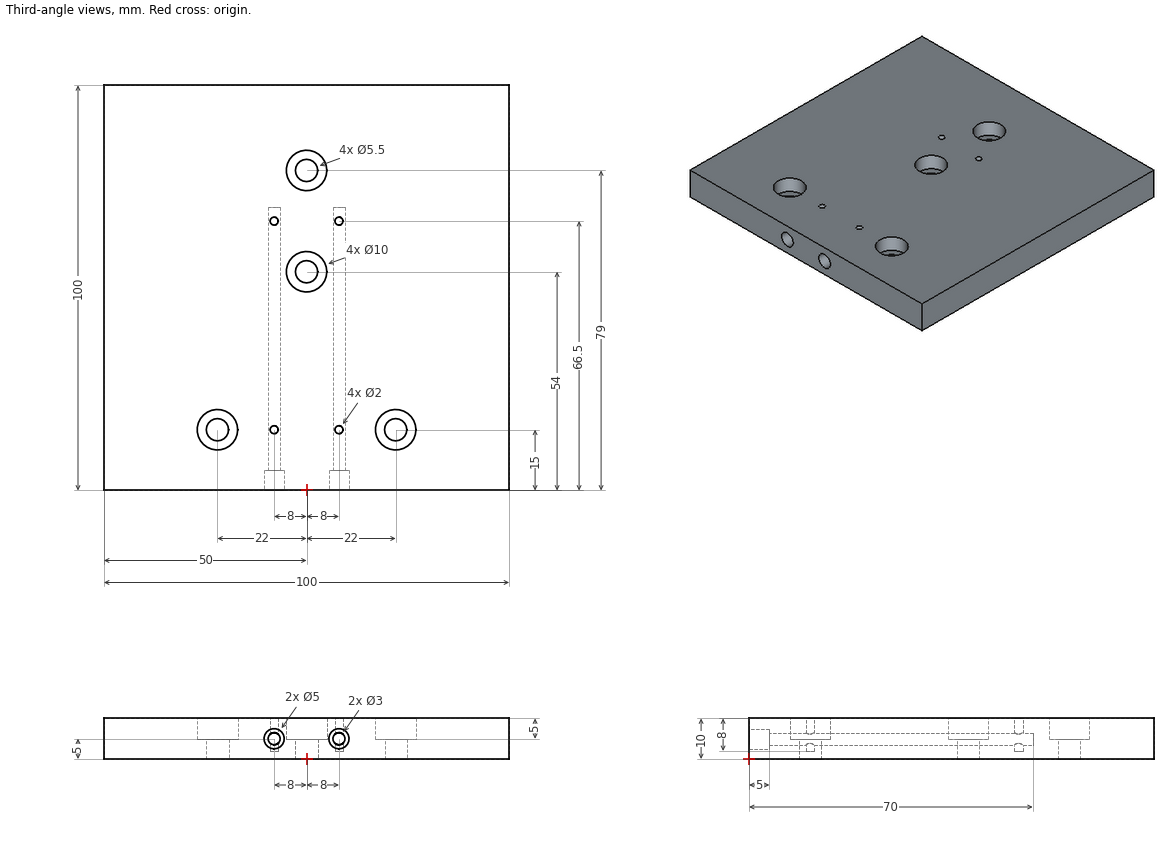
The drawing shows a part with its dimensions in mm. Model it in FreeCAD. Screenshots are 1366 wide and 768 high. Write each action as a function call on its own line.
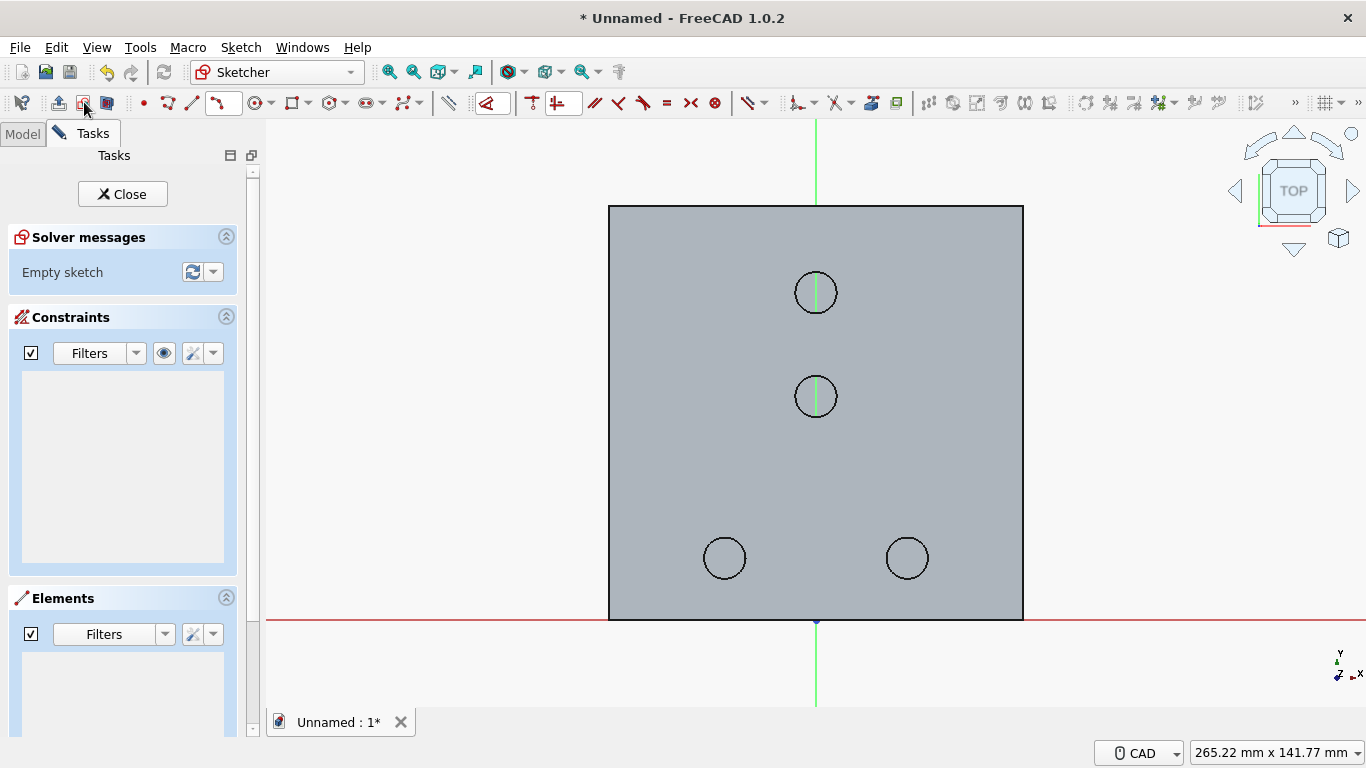
click(108, 104)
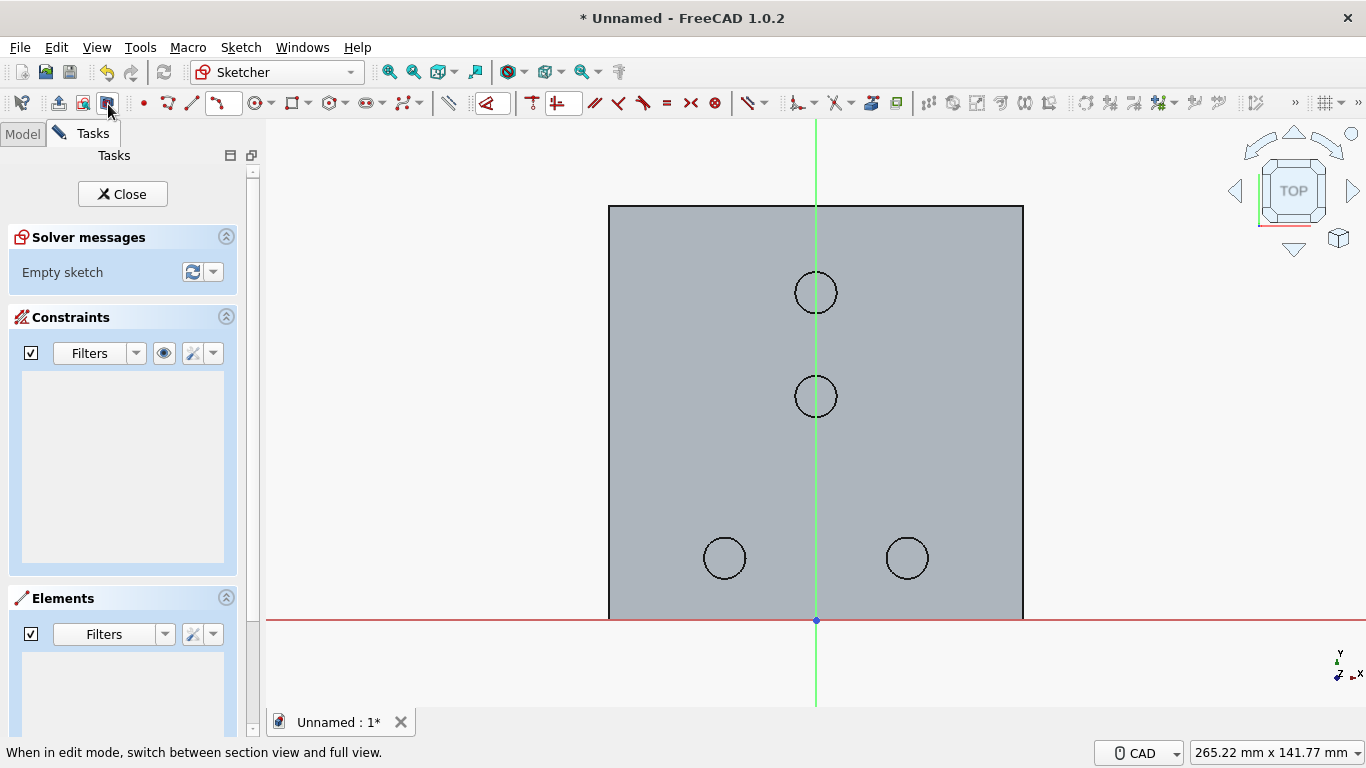
click(256, 104)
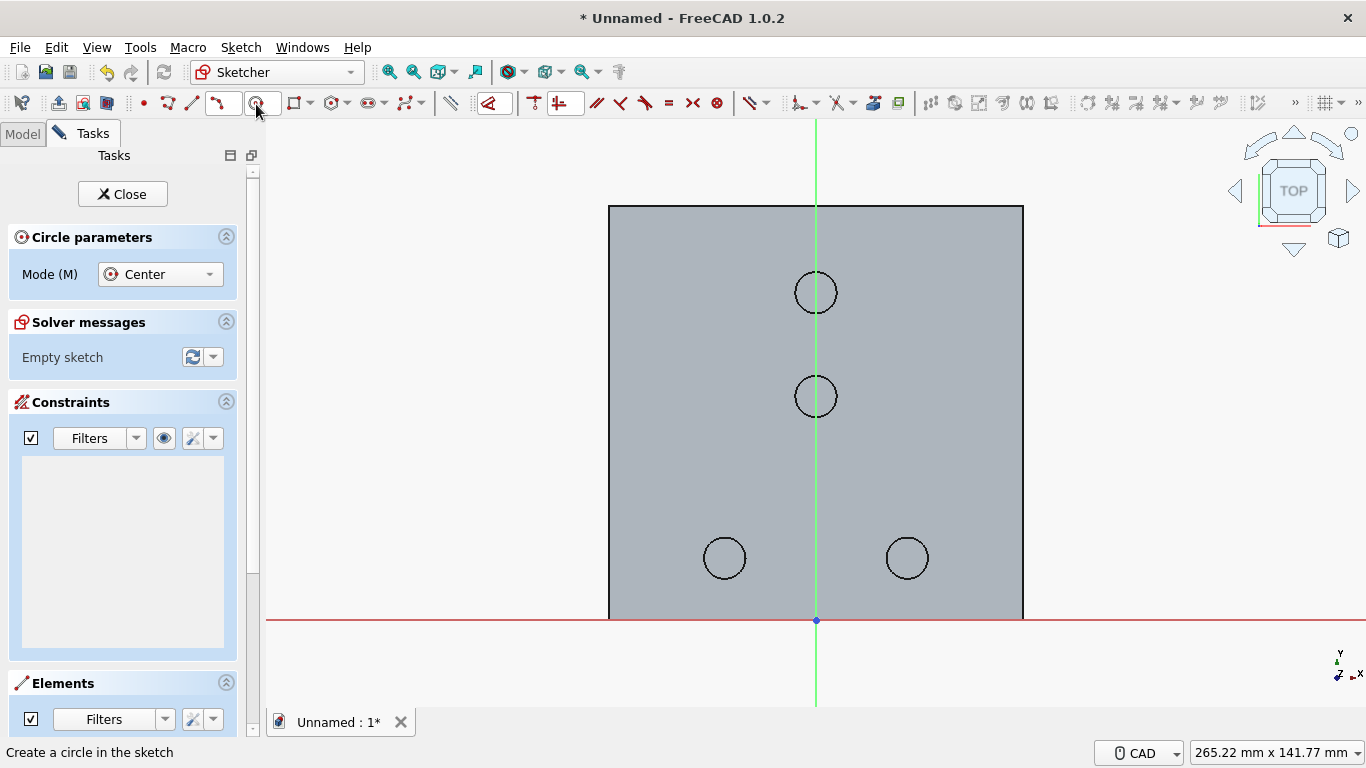
scroll(816, 293, up, 4)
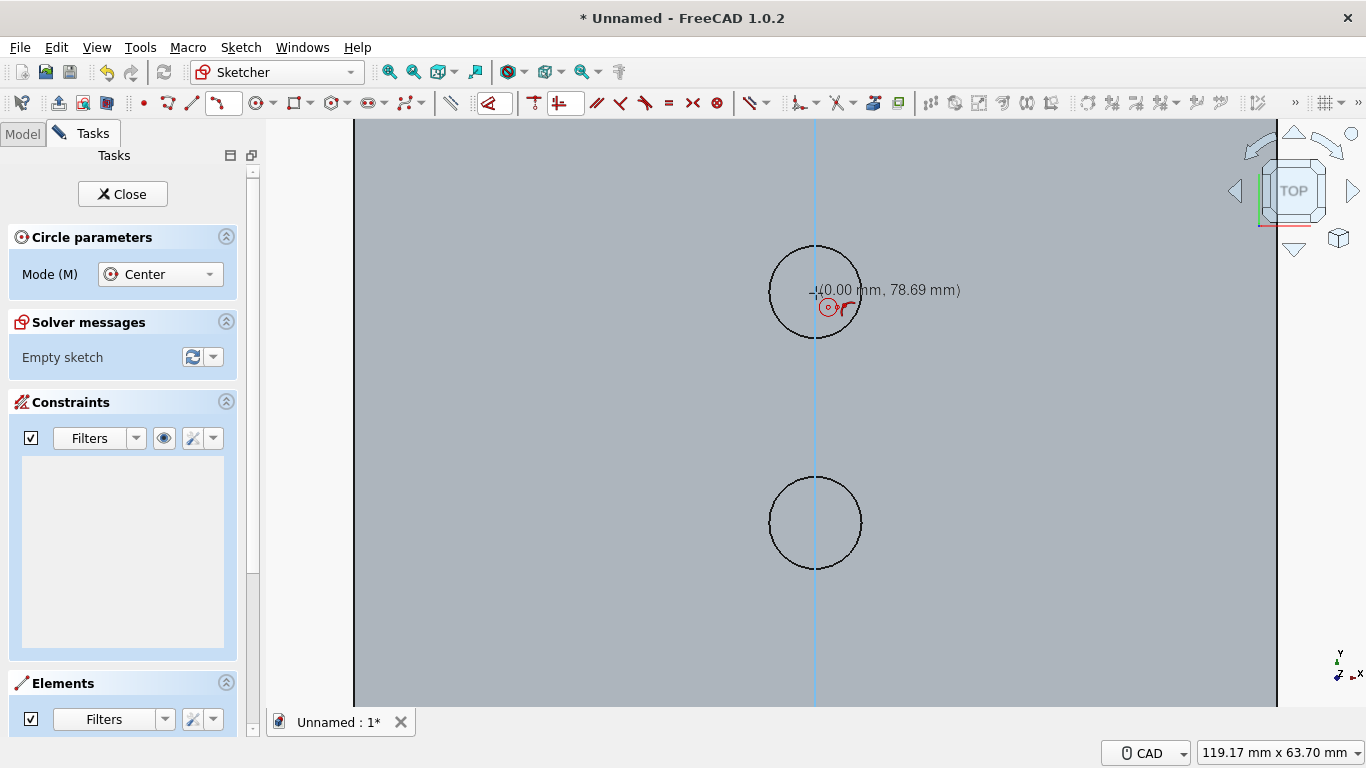
click(815, 292)
click(833, 274)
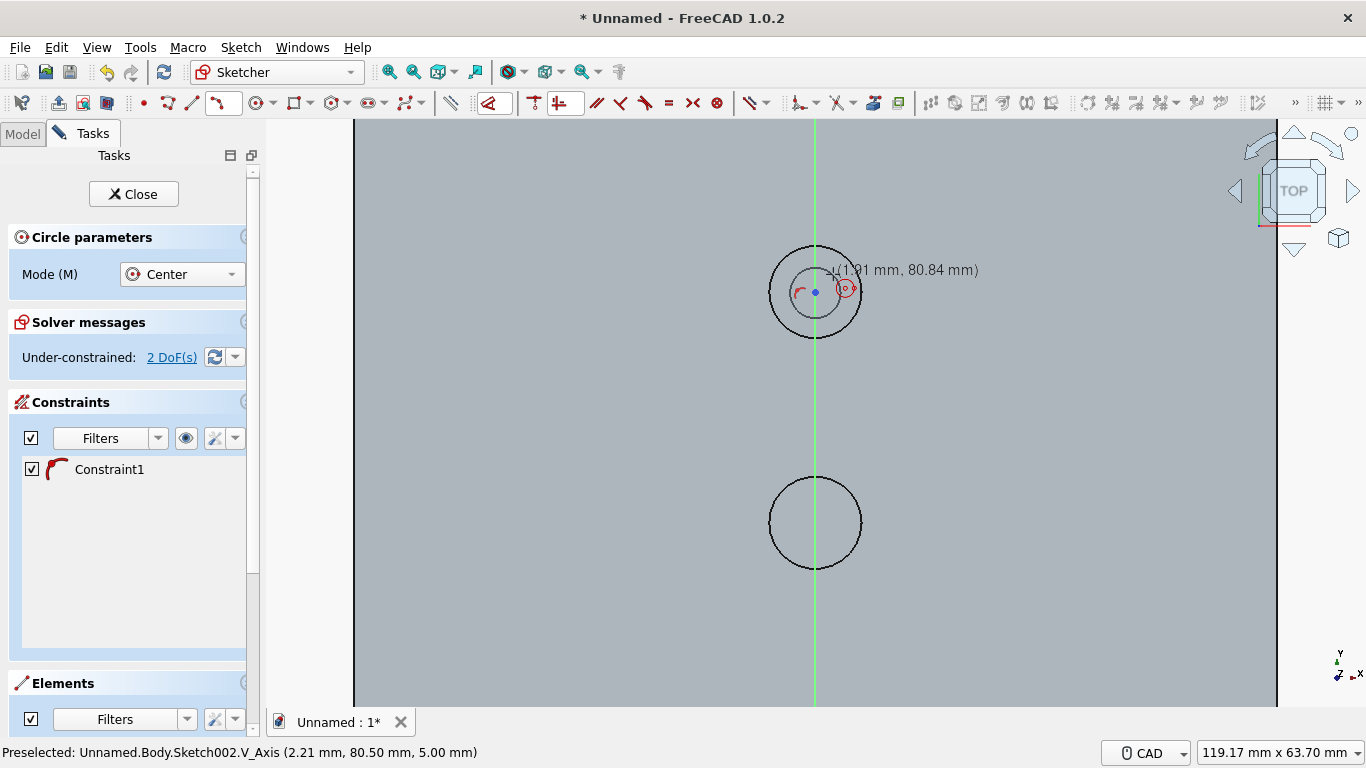
click(815, 523)
click(833, 505)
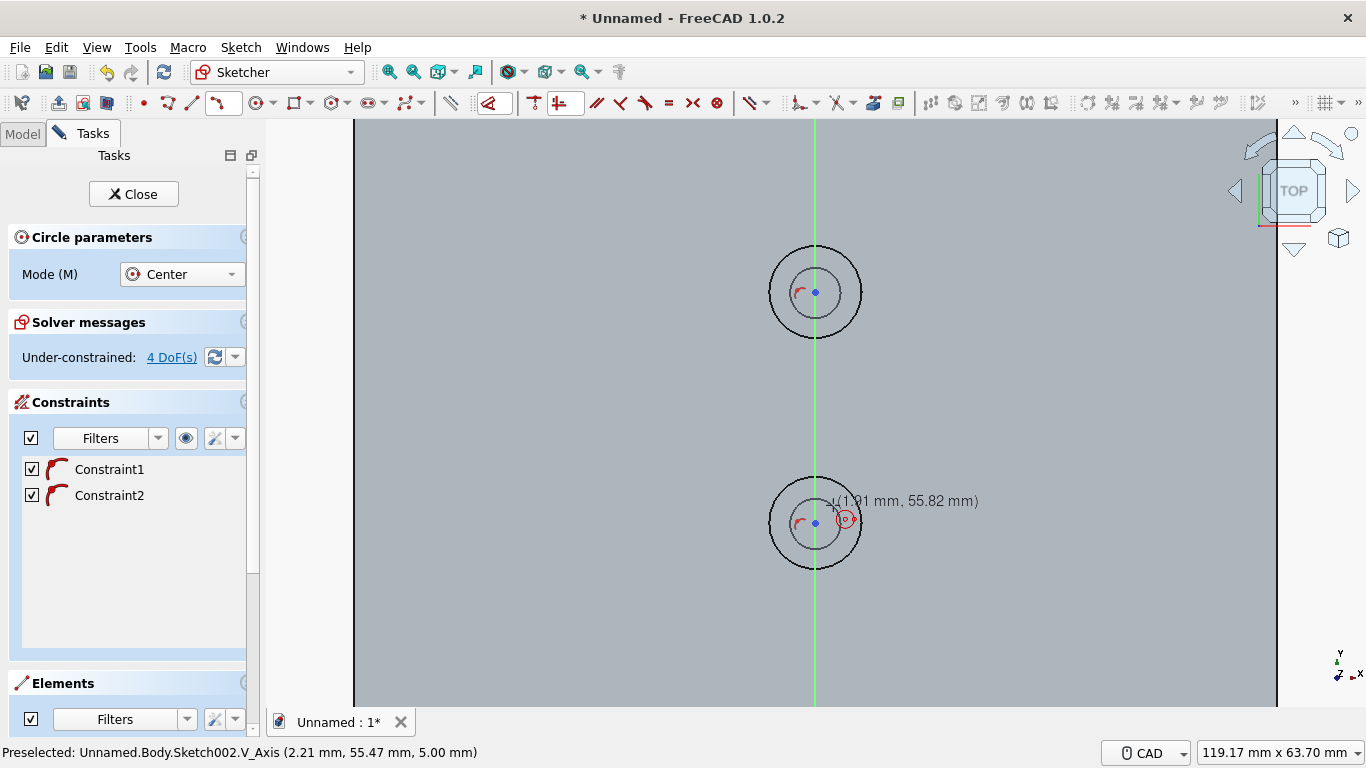
scroll(665, 147, down, 3)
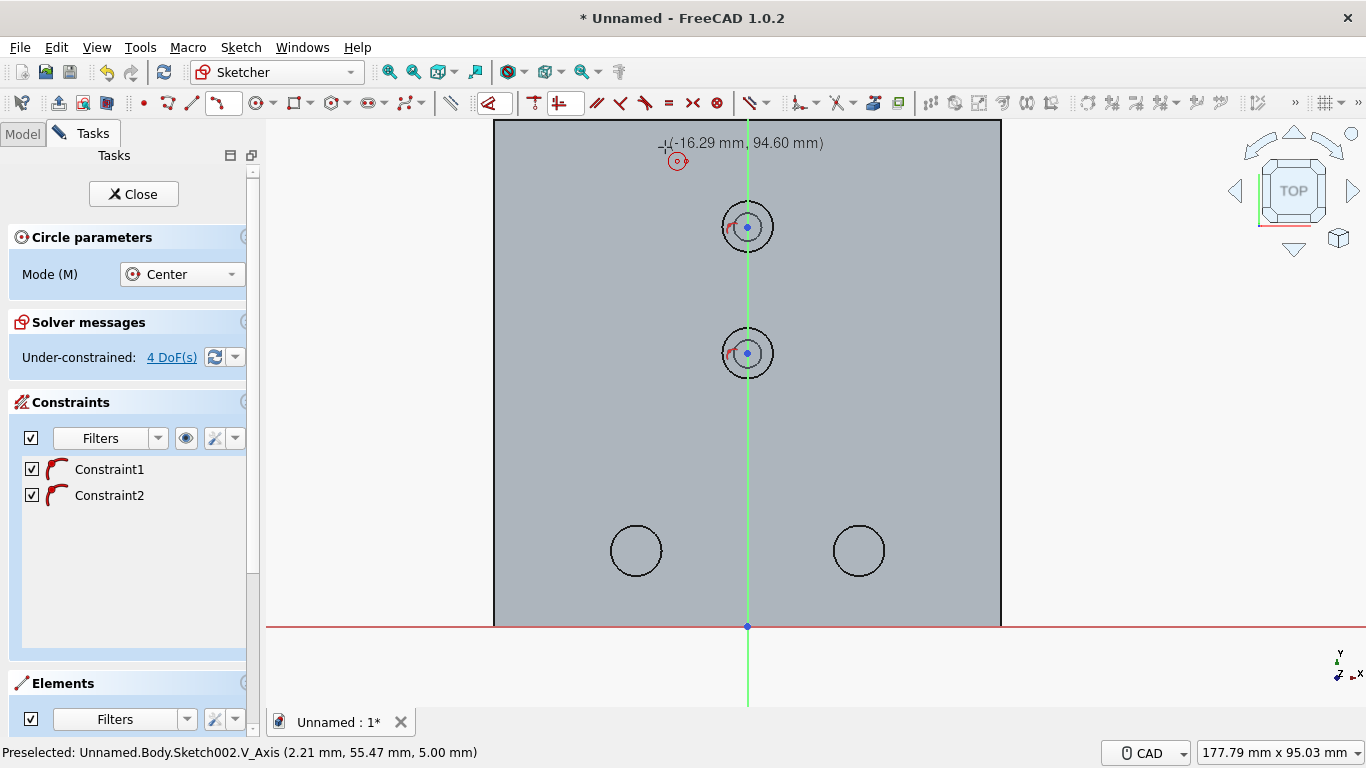
scroll(859, 551, up, 3)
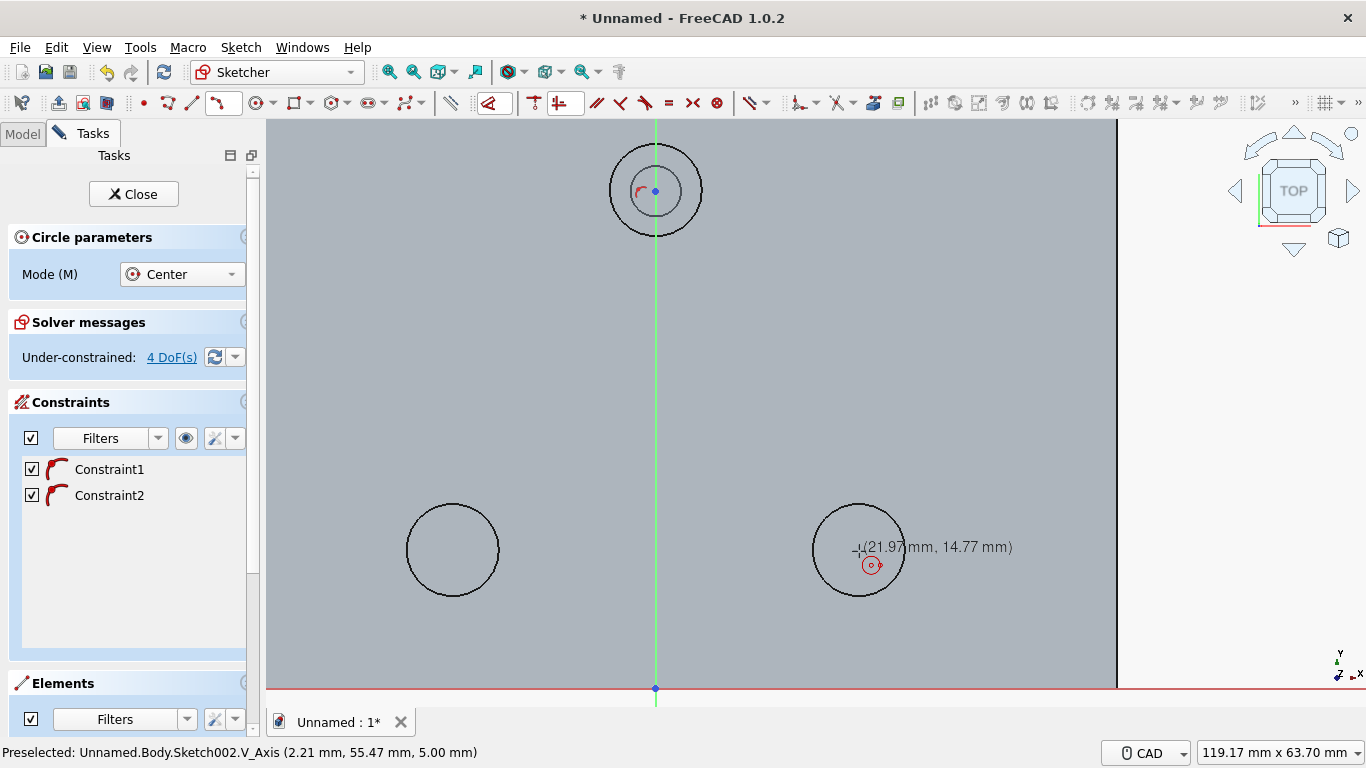
click(859, 550)
click(877, 532)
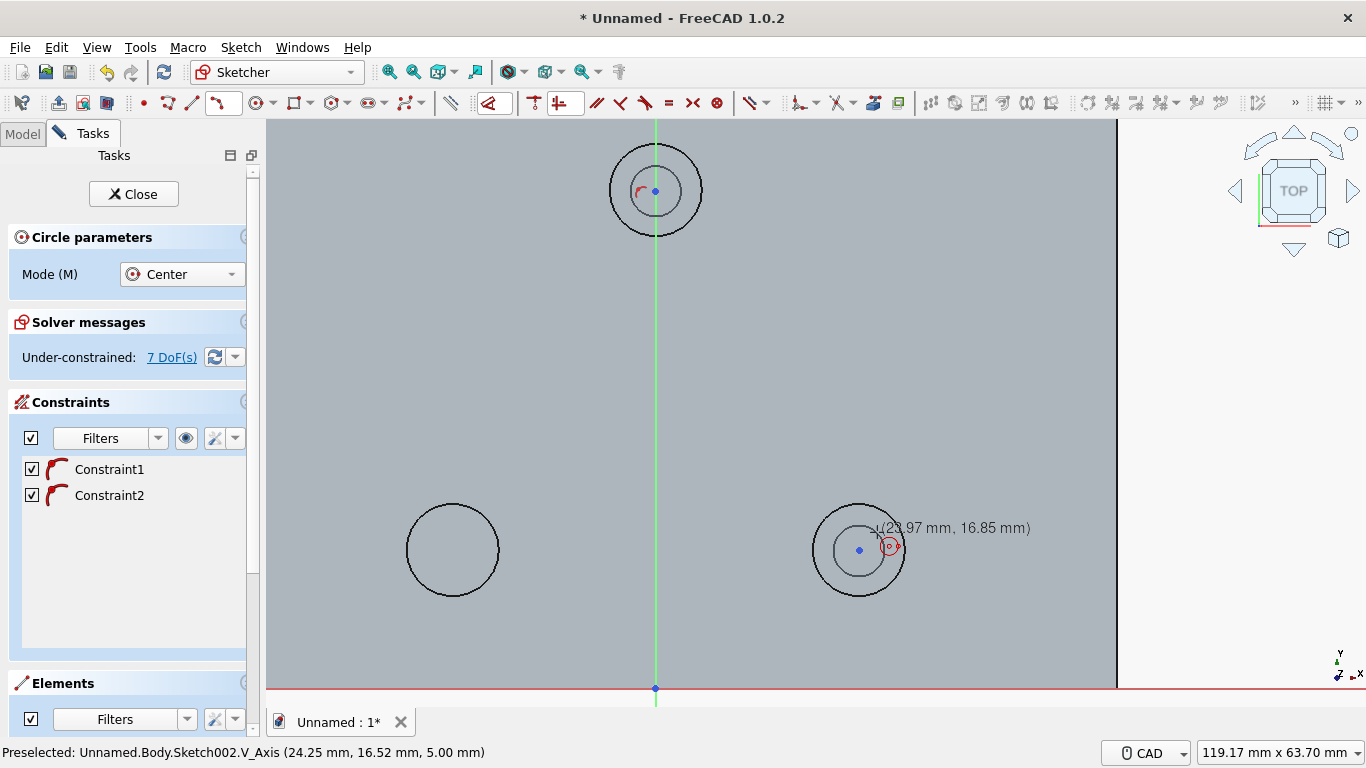
click(453, 550)
click(471, 532)
key(Escape)